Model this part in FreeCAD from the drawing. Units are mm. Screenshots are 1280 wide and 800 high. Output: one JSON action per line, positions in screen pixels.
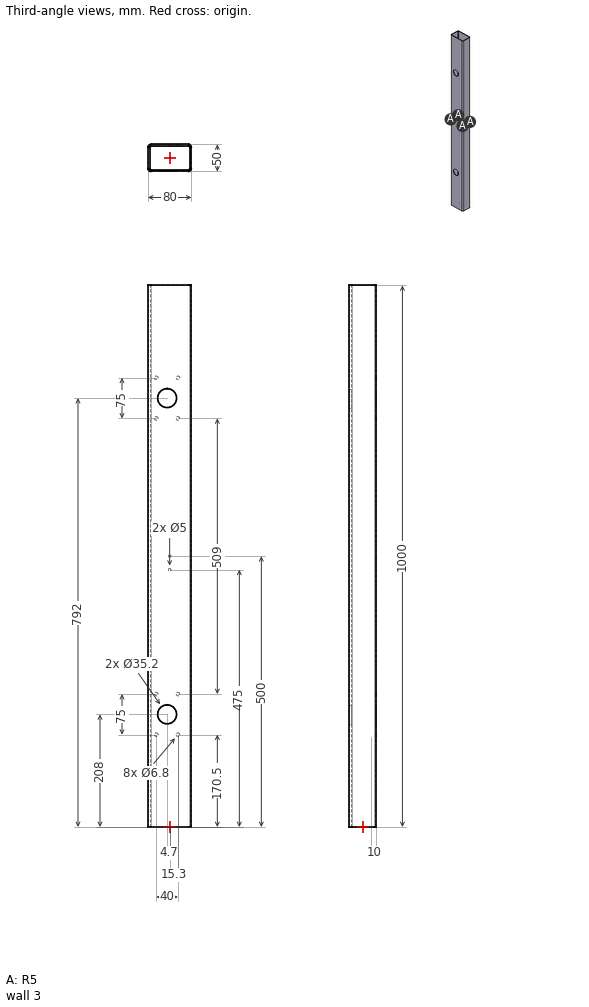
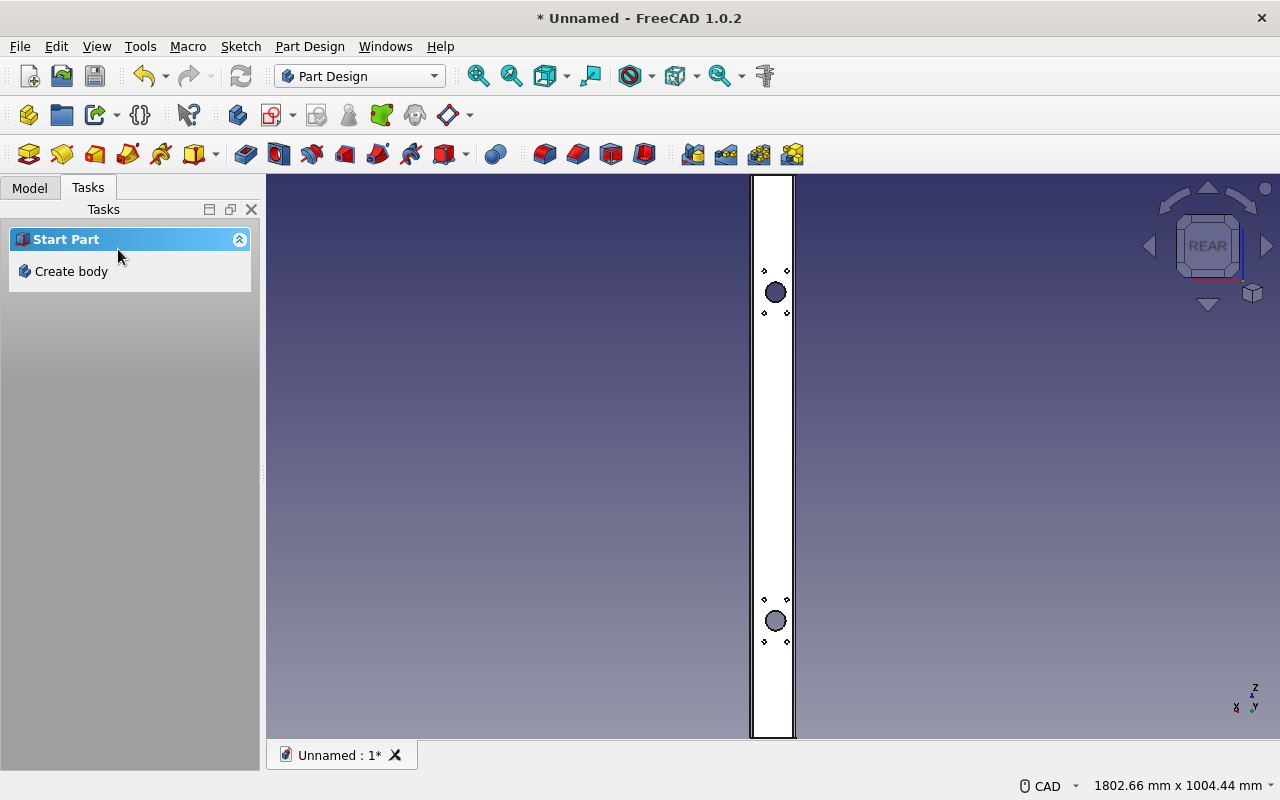
{"action": "left_click", "coordinate": [773, 214]}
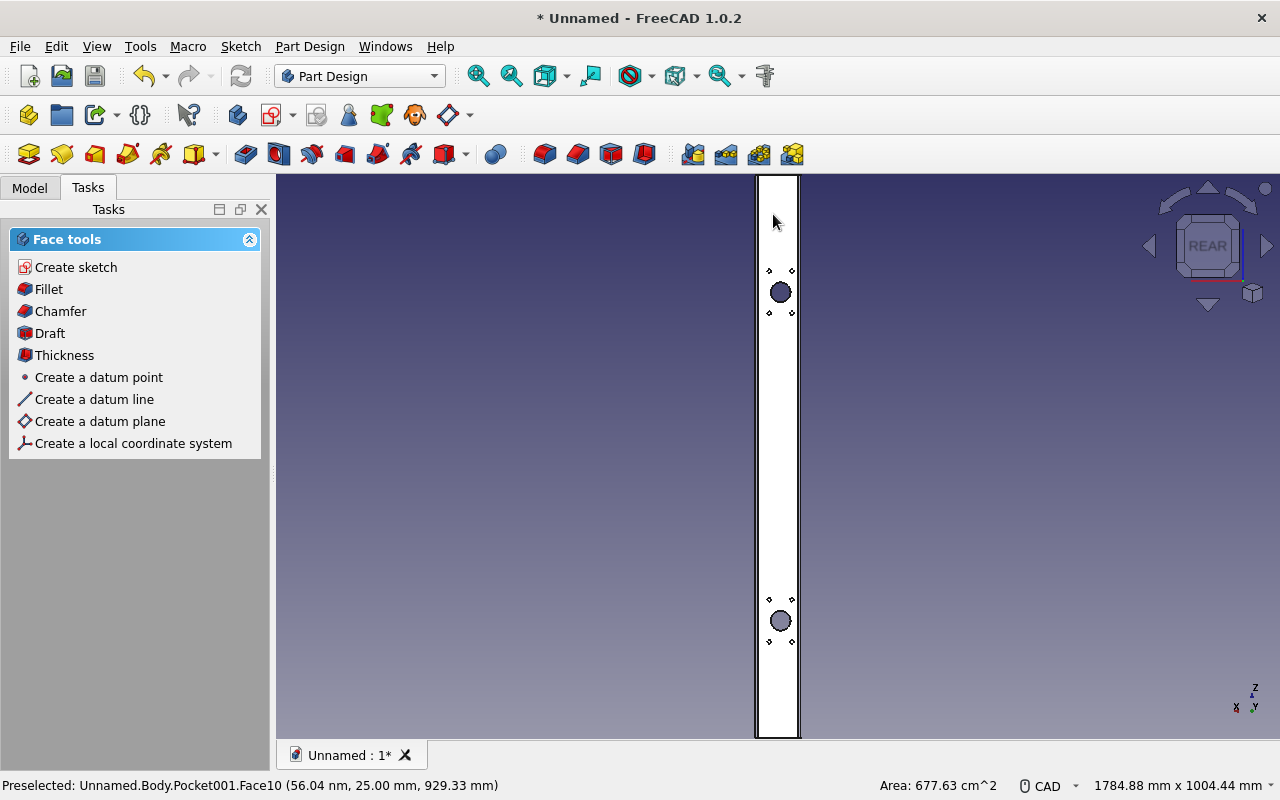
{"action": "left_click", "coordinate": [270, 116]}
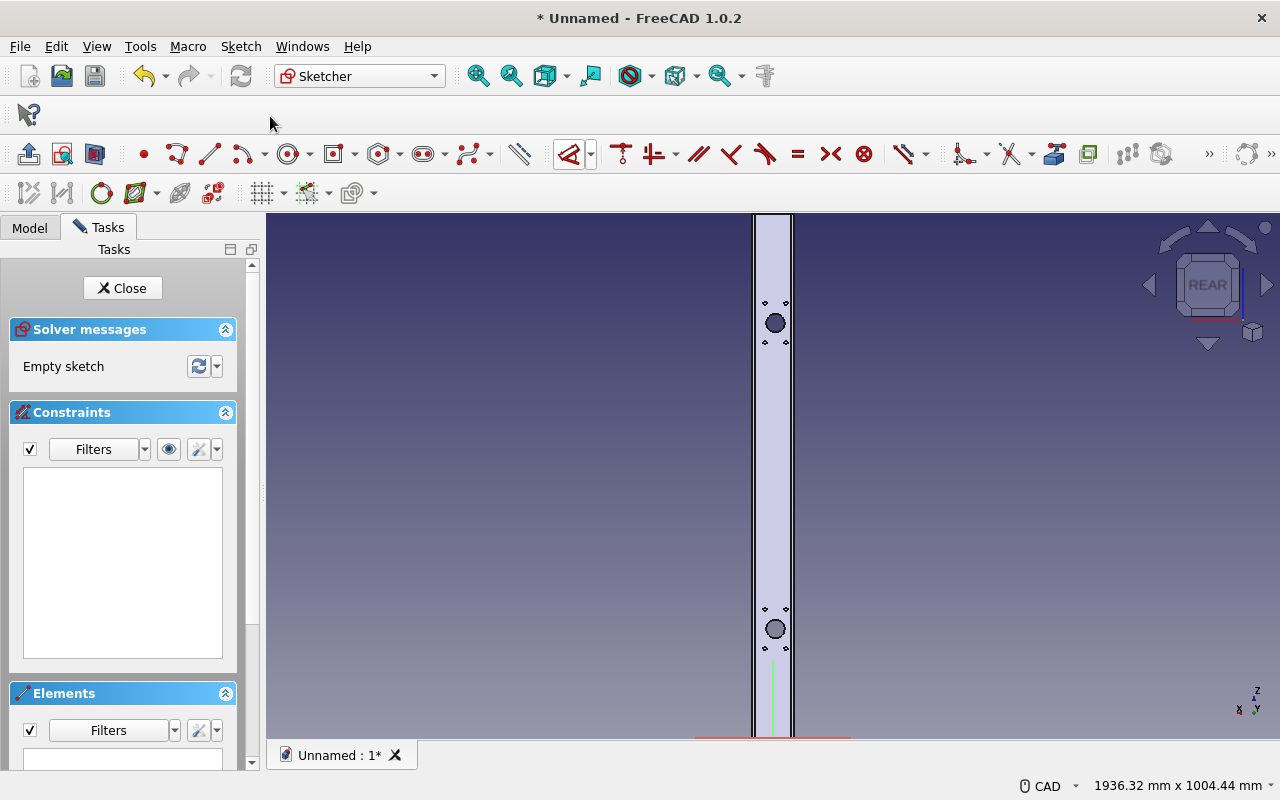
{"action": "scroll", "coordinate": [777, 483], "scroll_direction": "up", "scroll_amount": 15}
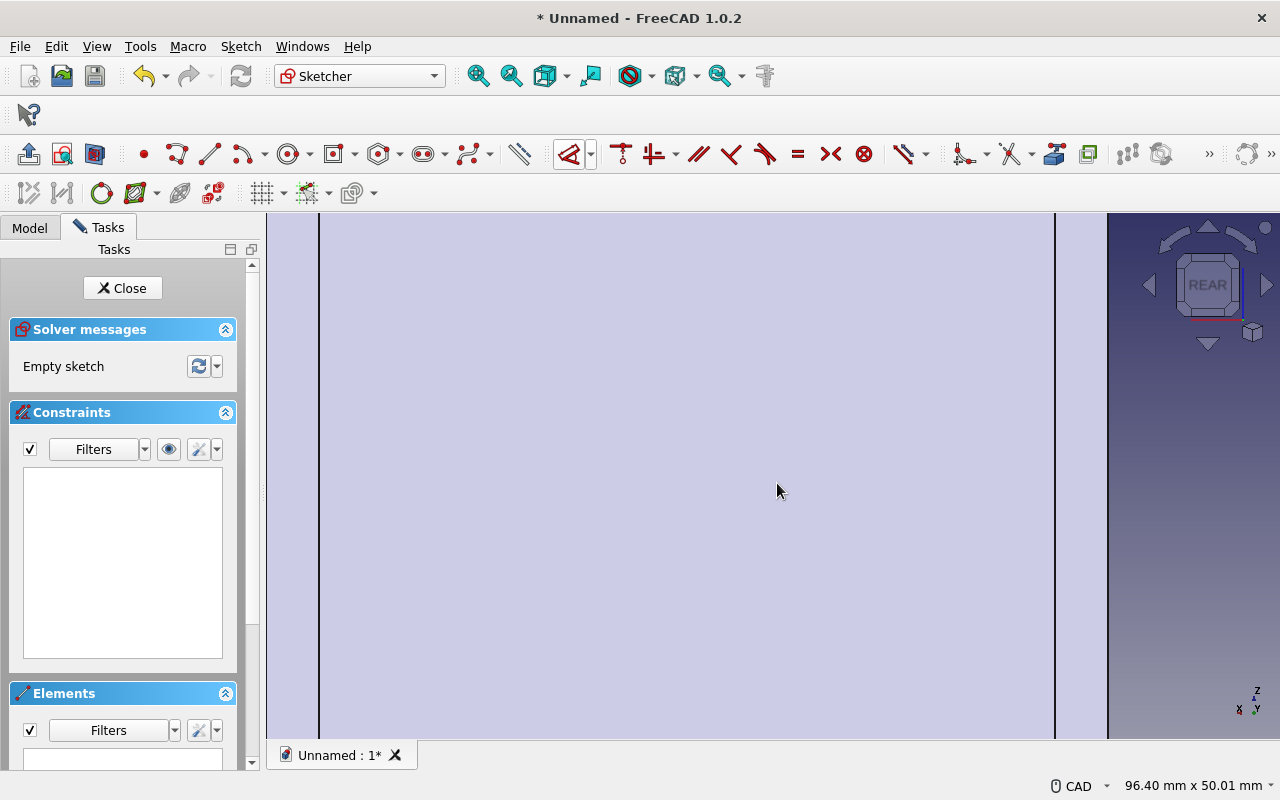
{"action": "left_click", "coordinate": [288, 154]}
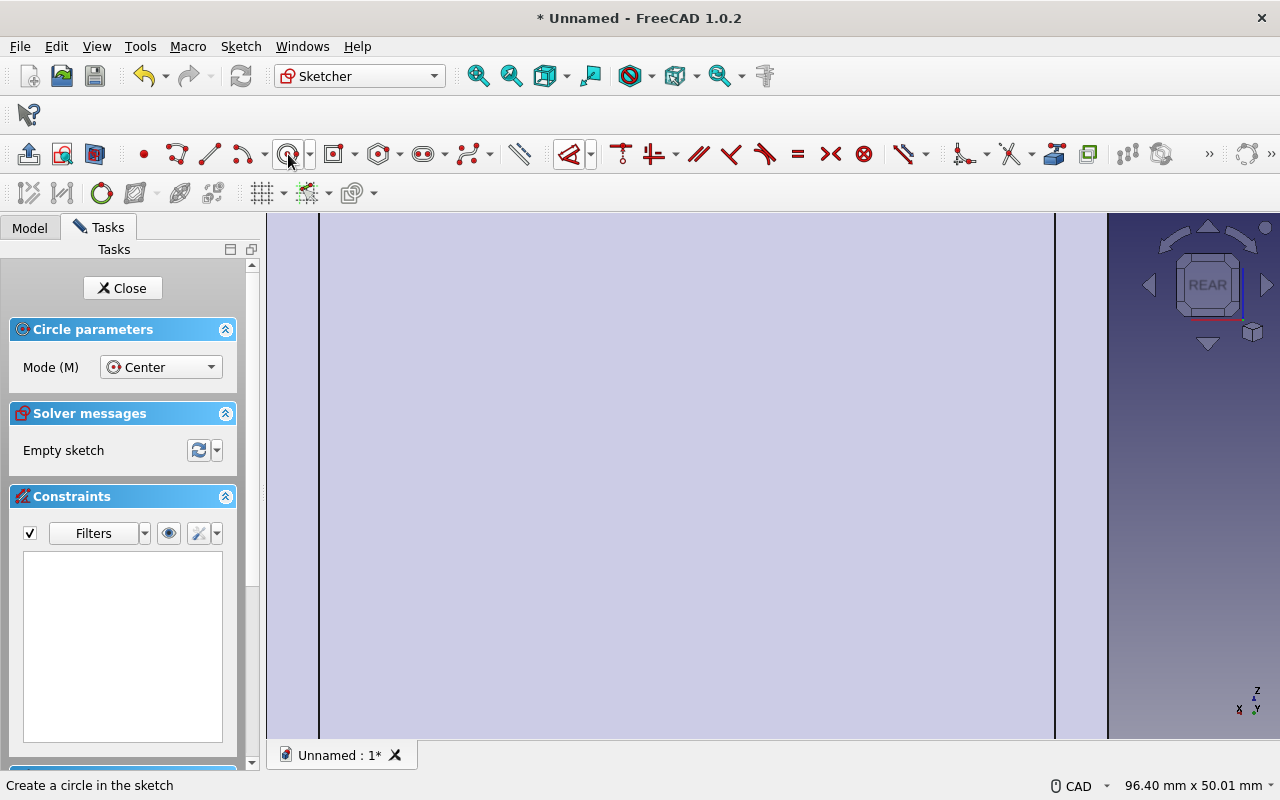
{"action": "left_click", "coordinate": [687, 596]}
{"action": "mouse_move", "coordinate": [706, 577]}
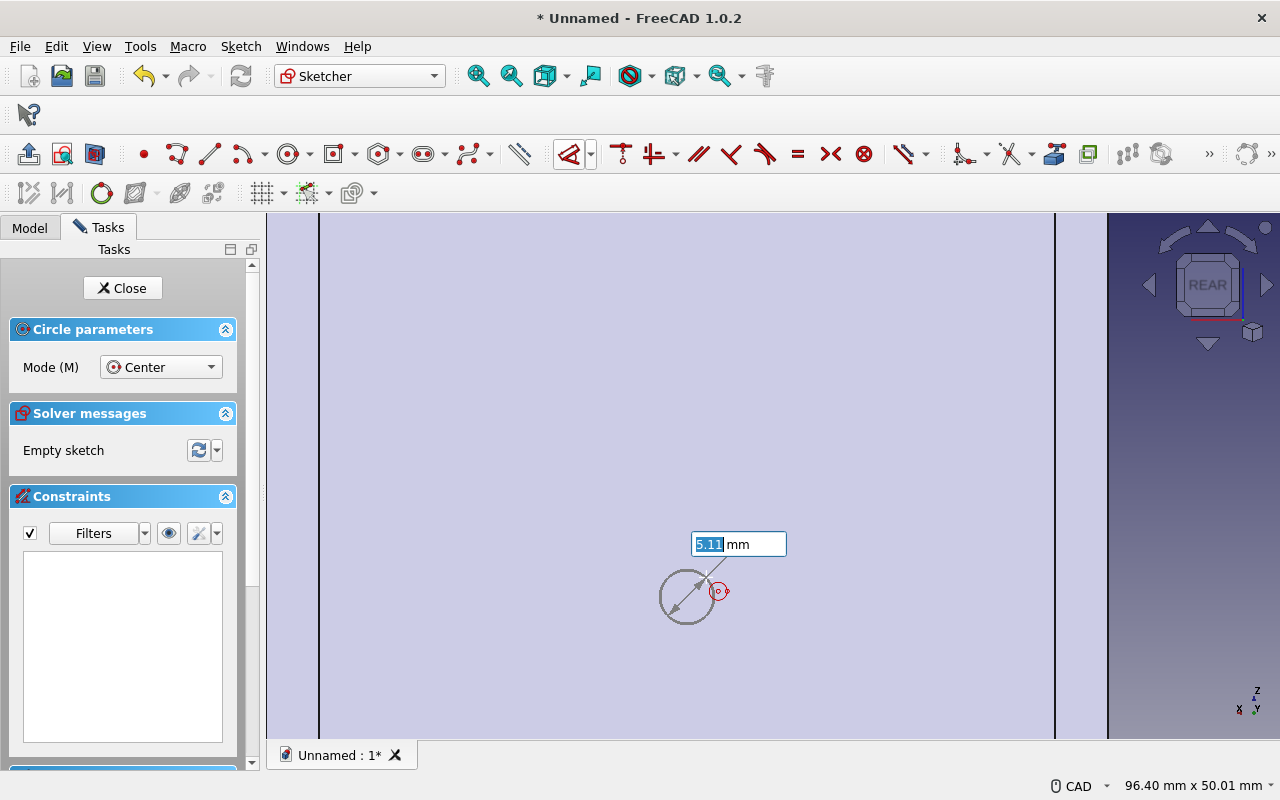
{"action": "type", "text": "5"}
{"action": "key", "text": "Return"}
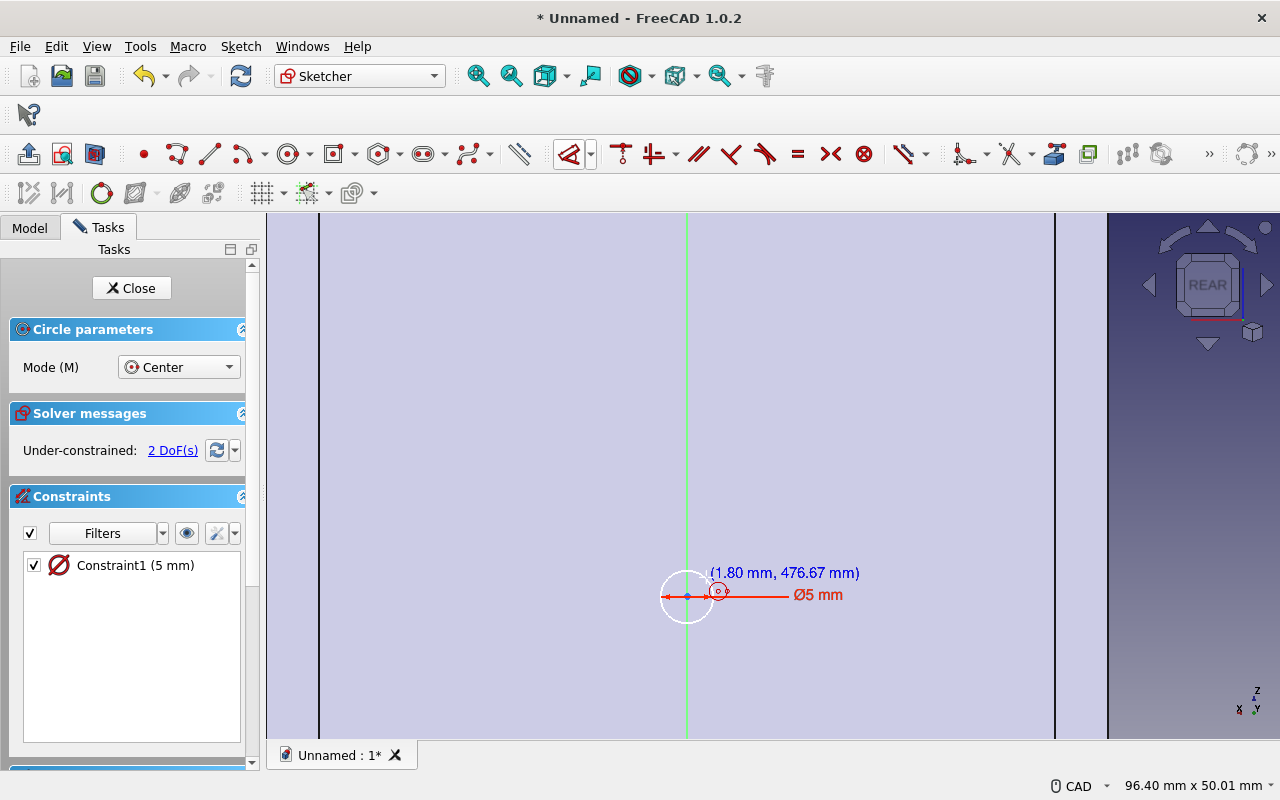
{"action": "left_click", "coordinate": [687, 333]}
{"action": "mouse_move", "coordinate": [706, 314]}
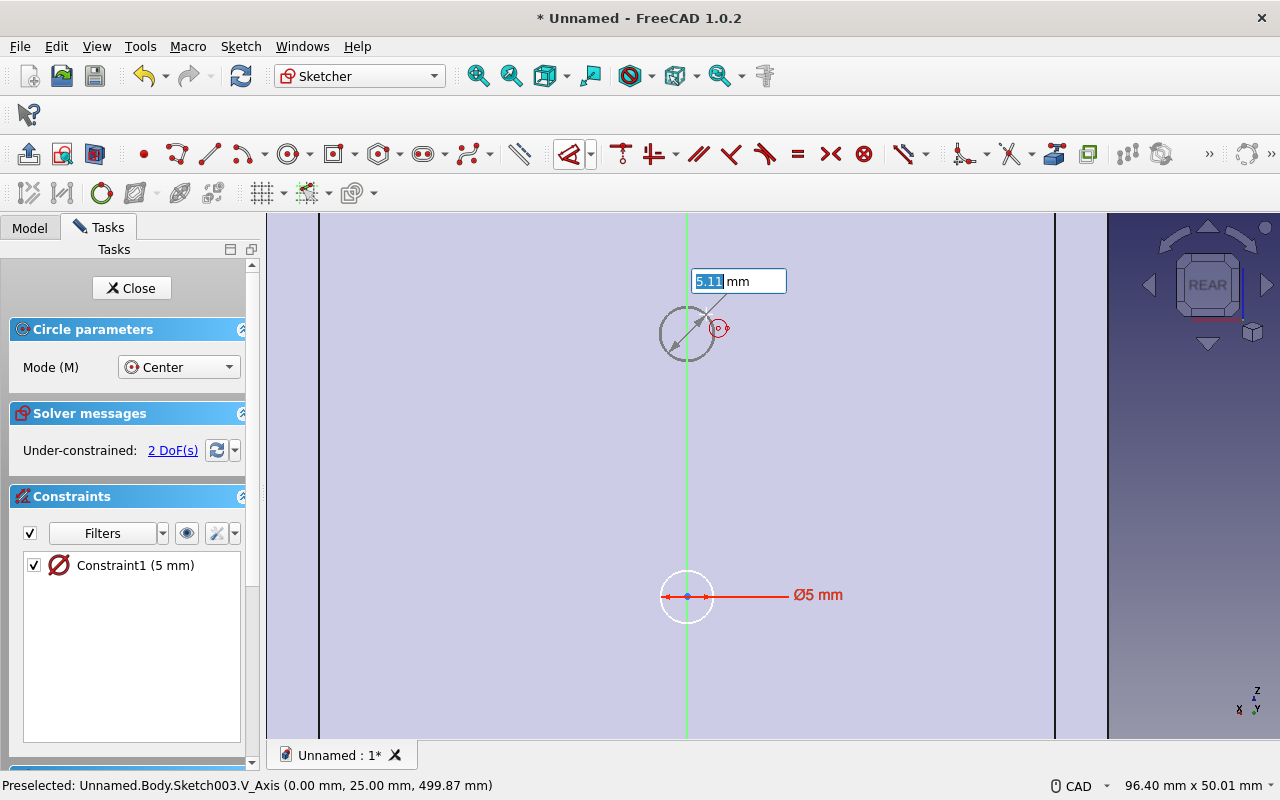
{"action": "type", "text": "5"}
{"action": "key", "text": "Return"}
{"action": "key", "text": "Escape"}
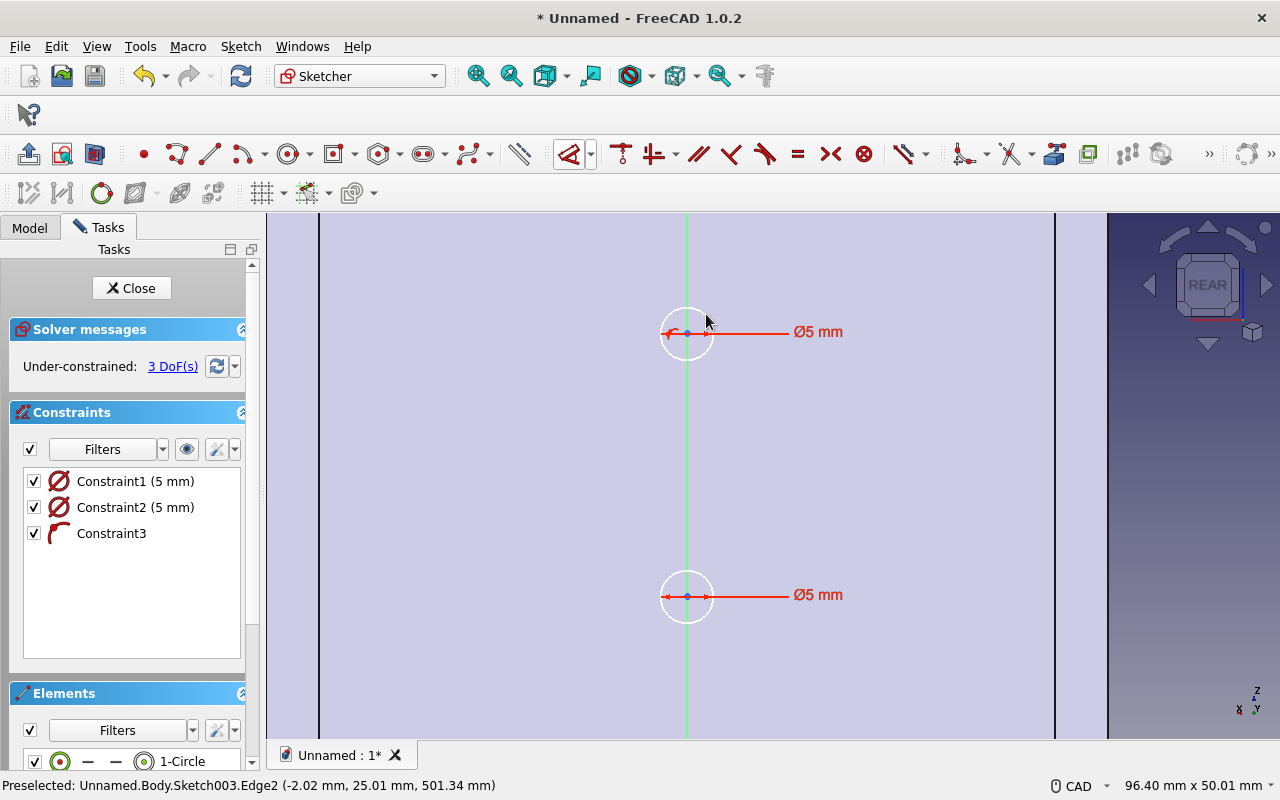
{"action": "left_click", "coordinate": [687, 597]}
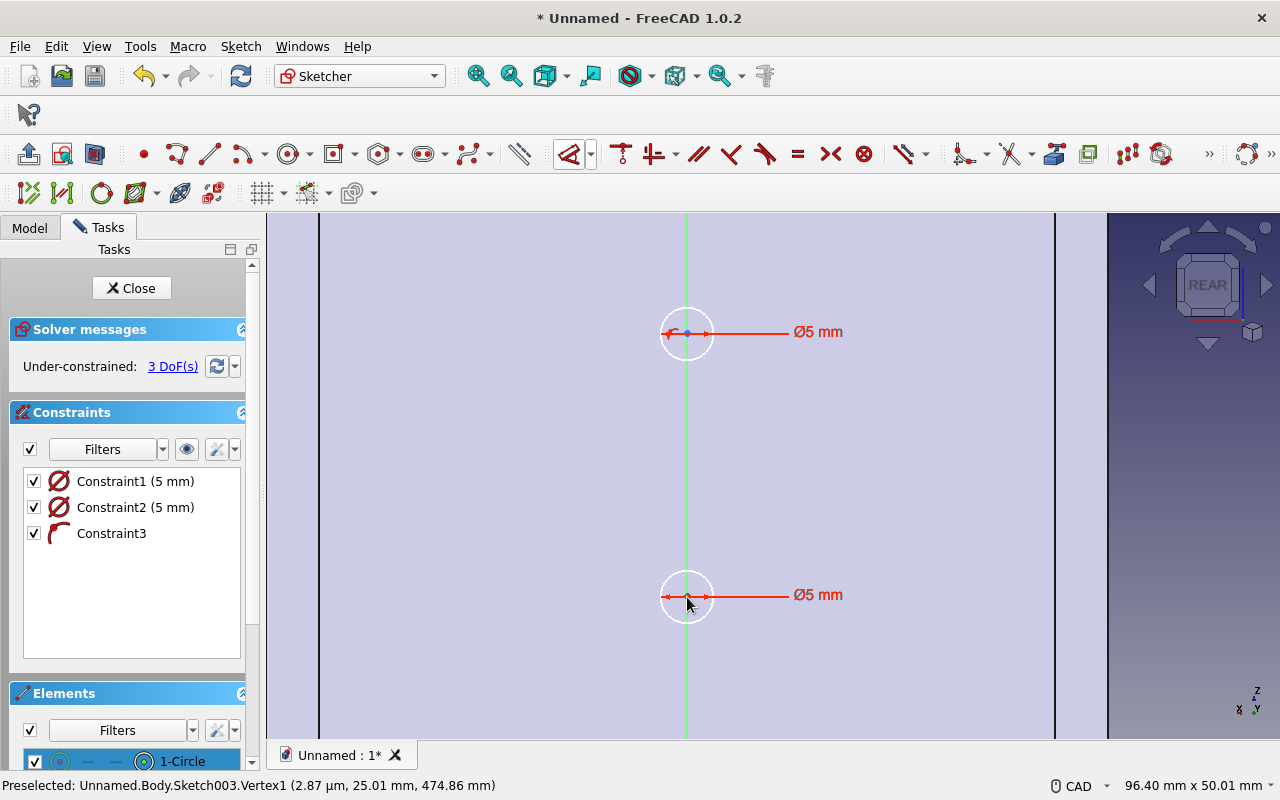
{"action": "left_click", "coordinate": [687, 677]}